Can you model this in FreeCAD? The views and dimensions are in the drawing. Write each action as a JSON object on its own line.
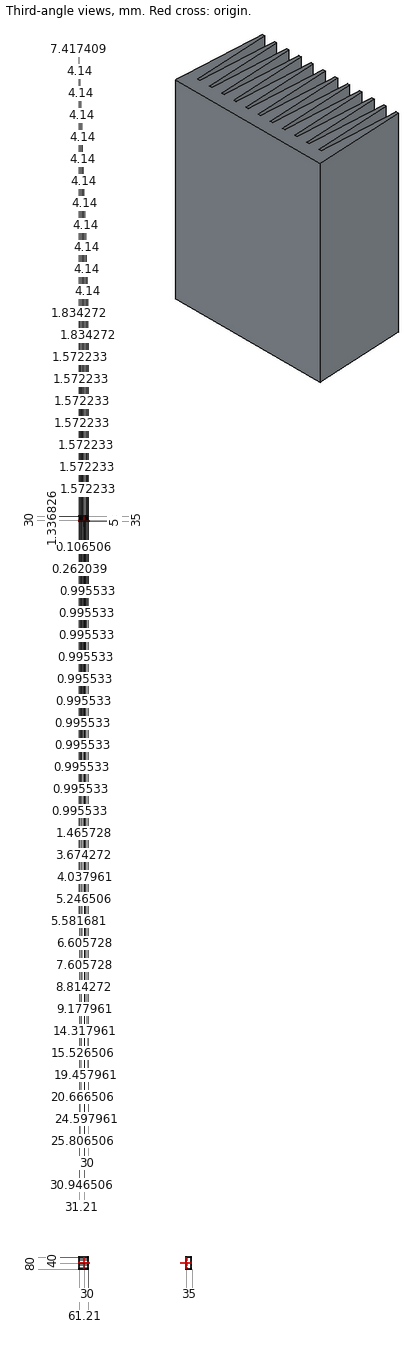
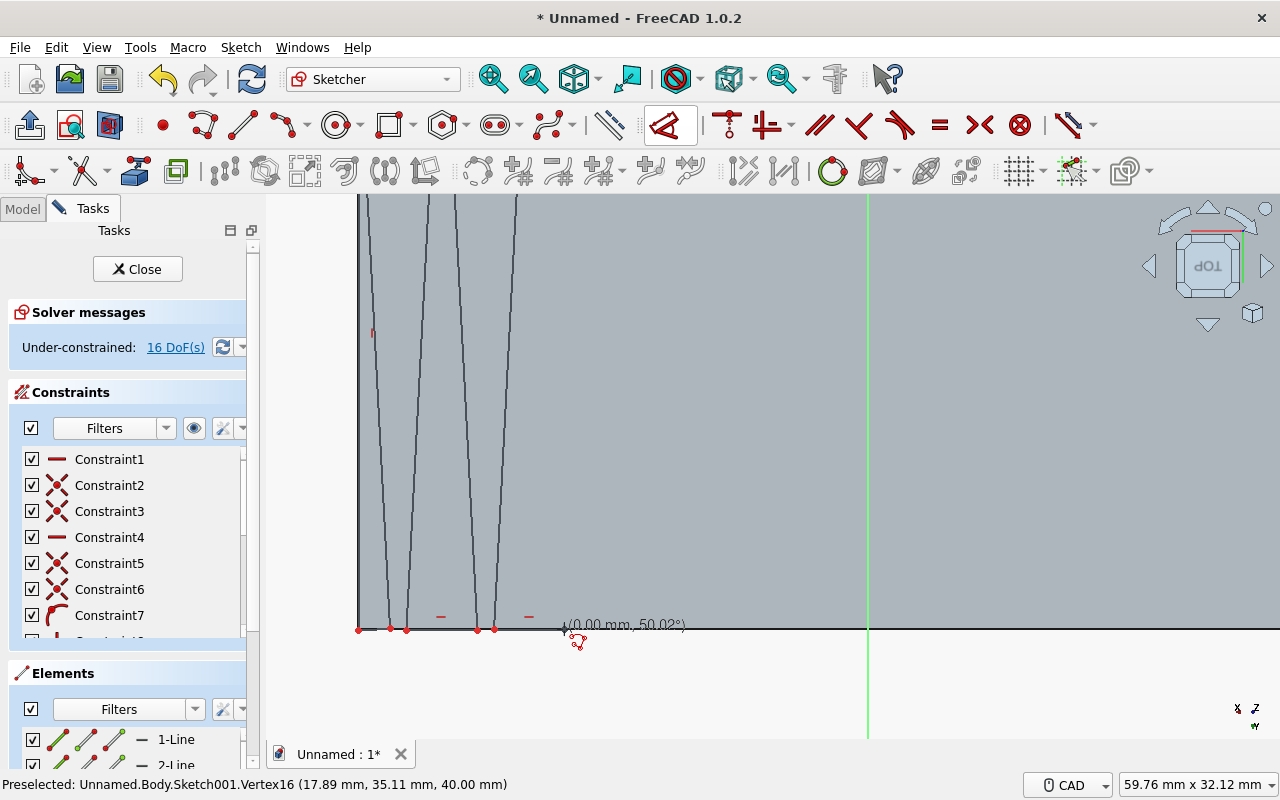
{"action": "scroll", "coordinate": [494, 630], "scroll_direction": "down", "scroll_amount": 3}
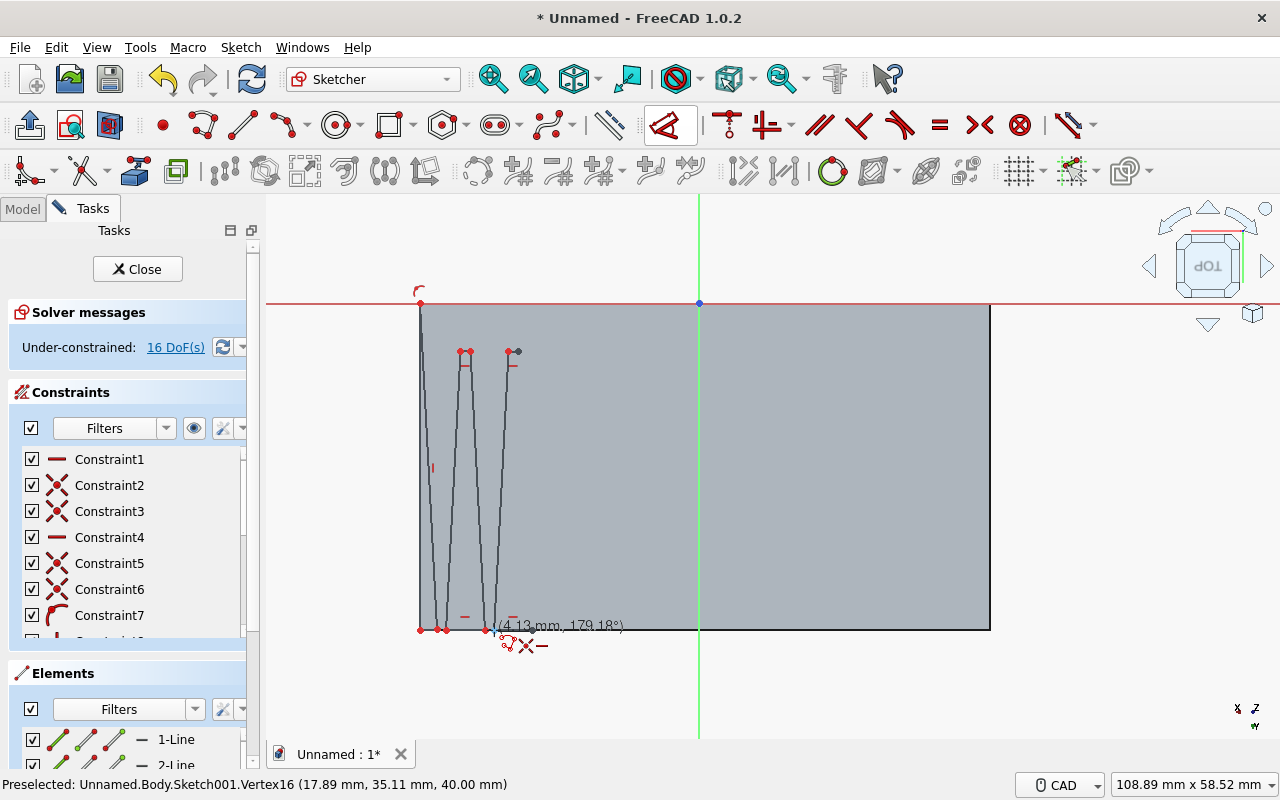
{"action": "scroll", "coordinate": [518, 351], "scroll_direction": "up", "scroll_amount": 7}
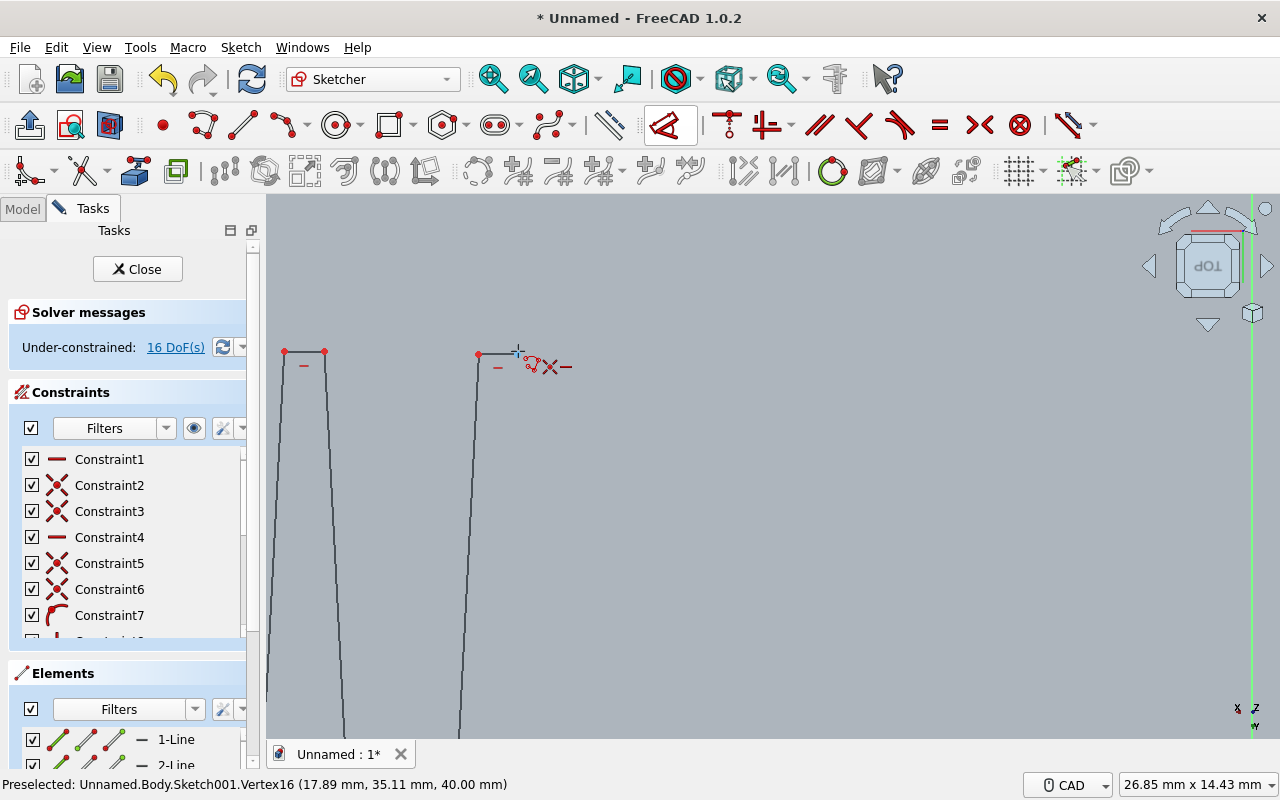
{"action": "left_click", "coordinate": [517, 354]}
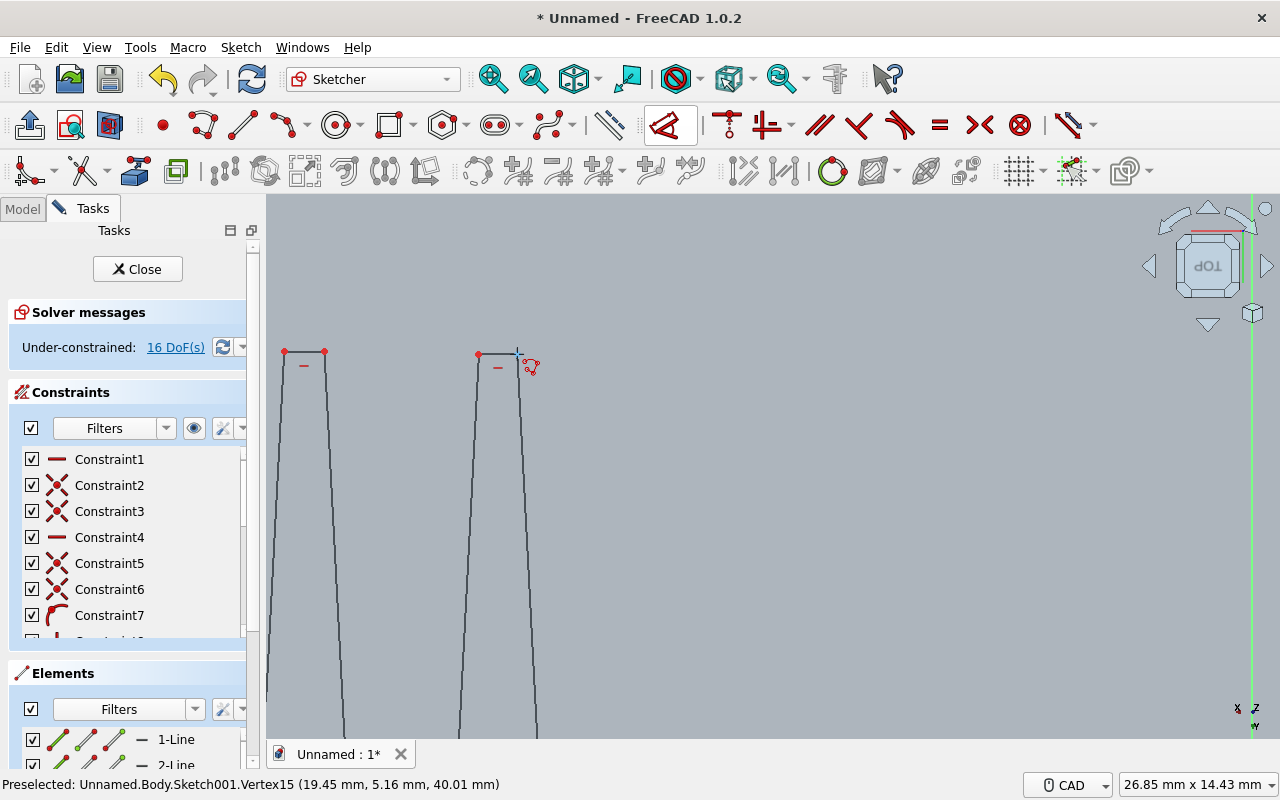
{"action": "scroll", "coordinate": [518, 351], "scroll_direction": "down", "scroll_amount": 7}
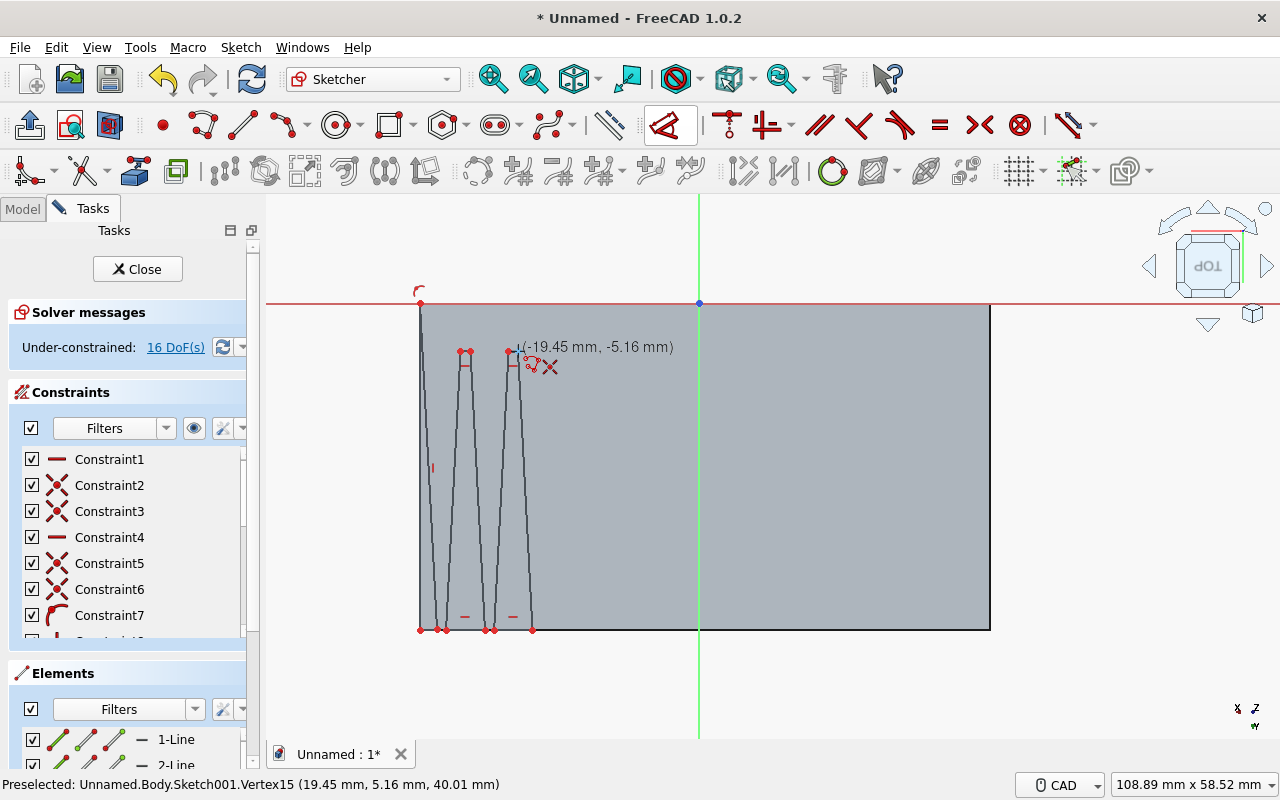
{"action": "left_click", "coordinate": [566, 351]}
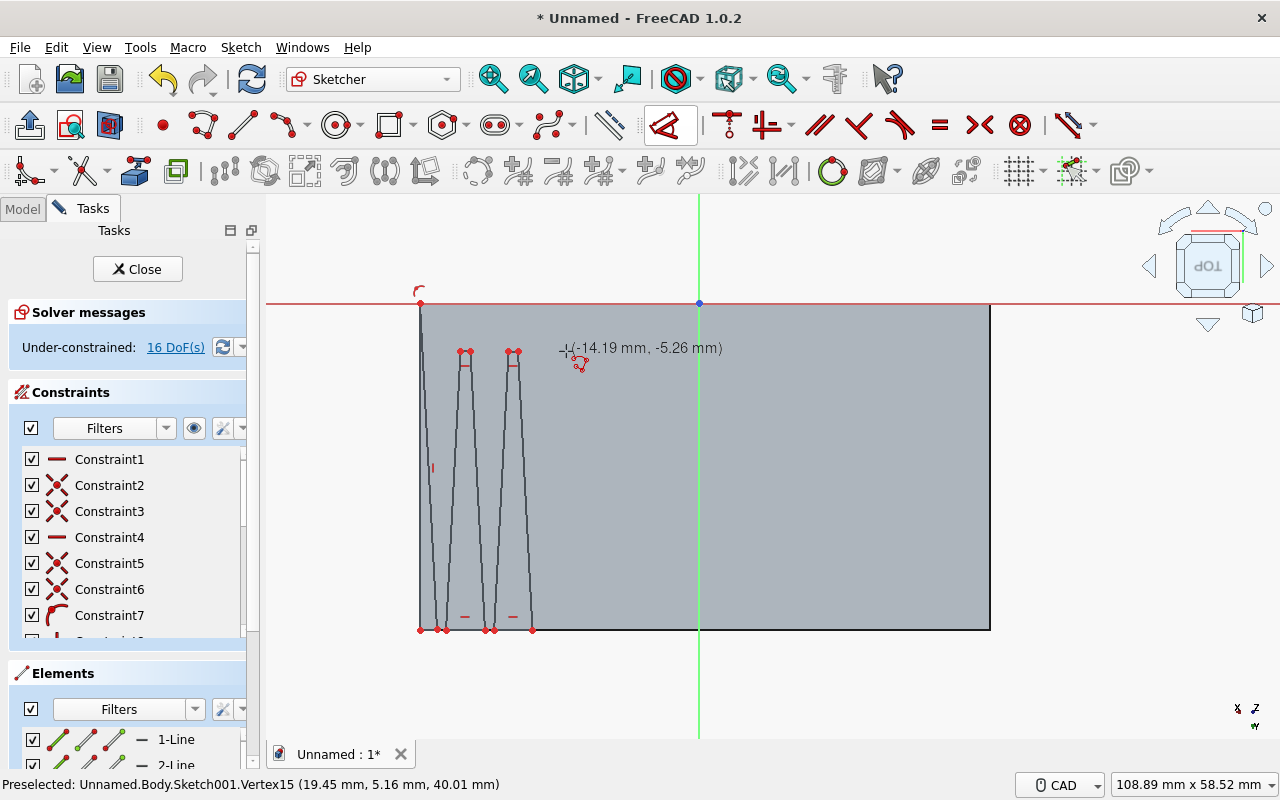
{"action": "scroll", "coordinate": [556, 351], "scroll_direction": "up", "scroll_amount": 3}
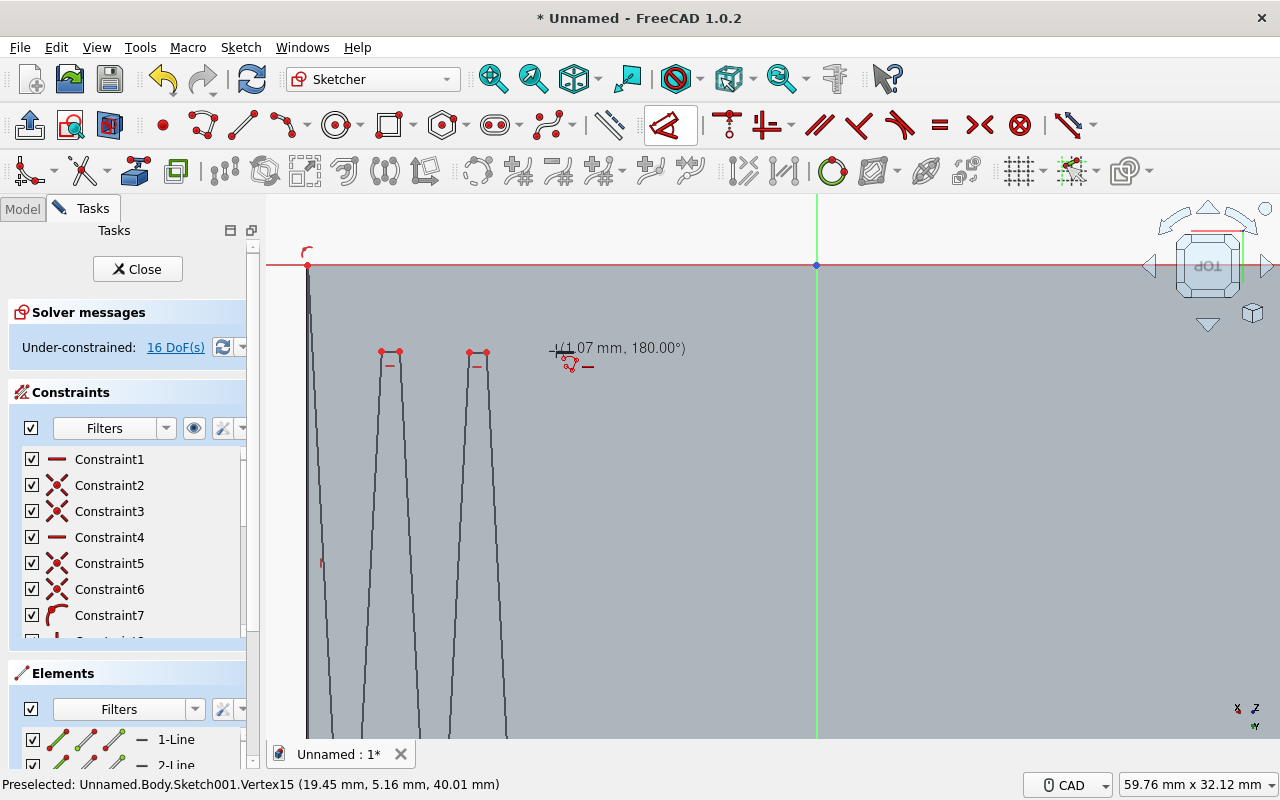
{"action": "left_click", "coordinate": [557, 351]}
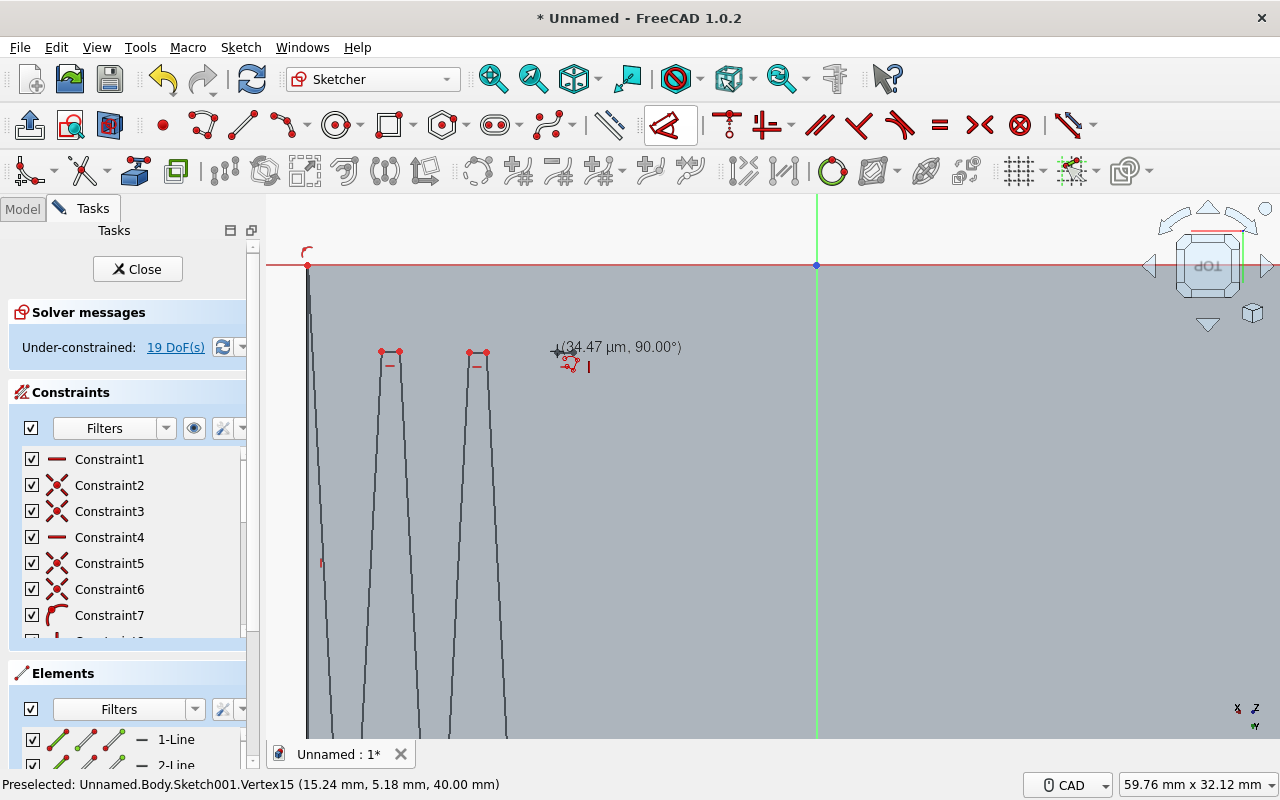
{"action": "scroll", "coordinate": [556, 350], "scroll_direction": "down", "scroll_amount": 3}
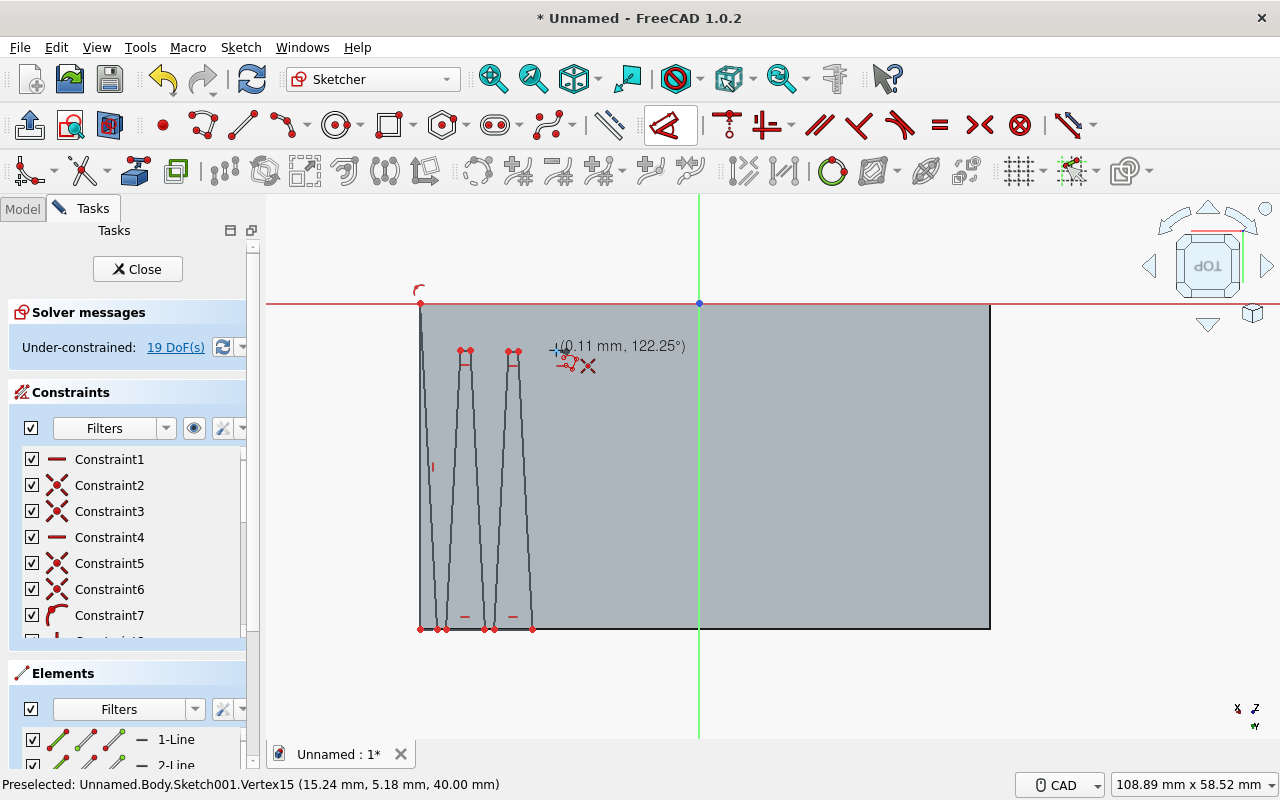
{"action": "scroll", "coordinate": [542, 629], "scroll_direction": "up", "scroll_amount": 3}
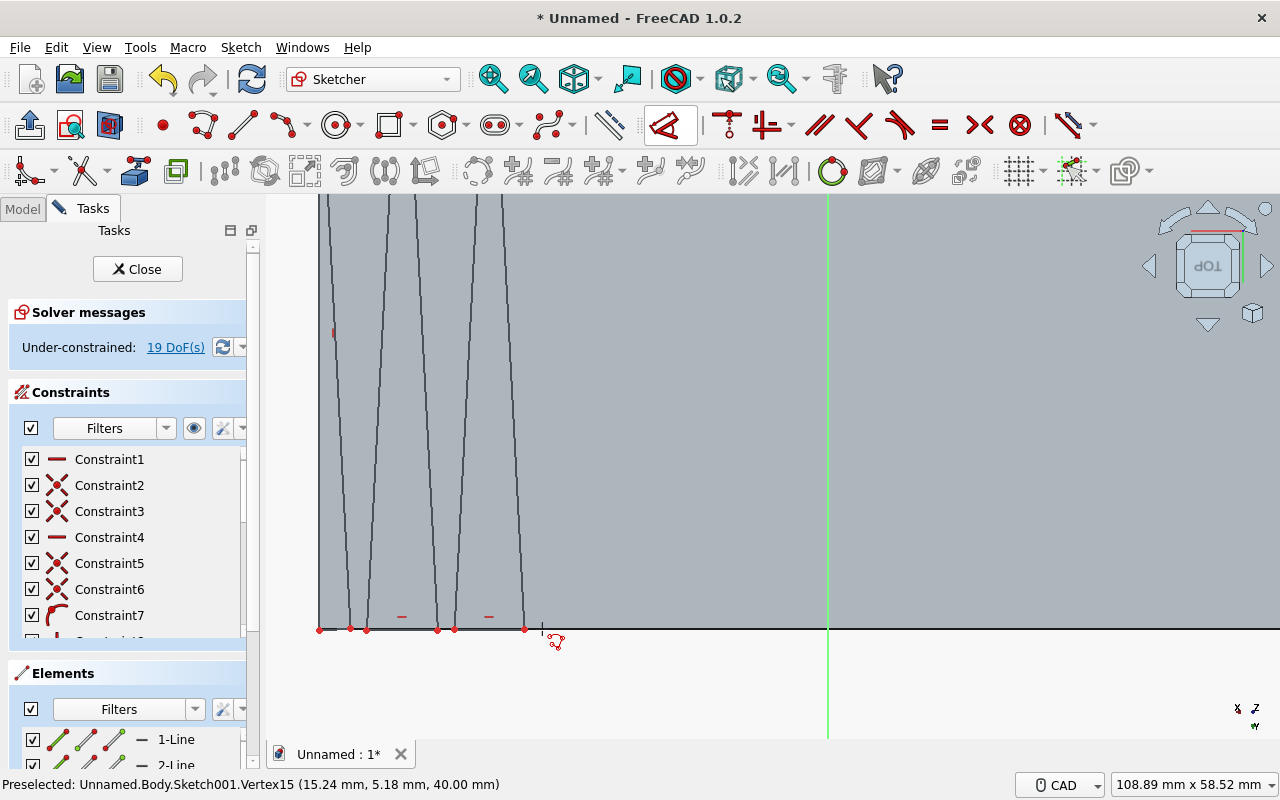
{"action": "left_click", "coordinate": [542, 629]}
{"action": "left_click", "coordinate": [612, 629]}